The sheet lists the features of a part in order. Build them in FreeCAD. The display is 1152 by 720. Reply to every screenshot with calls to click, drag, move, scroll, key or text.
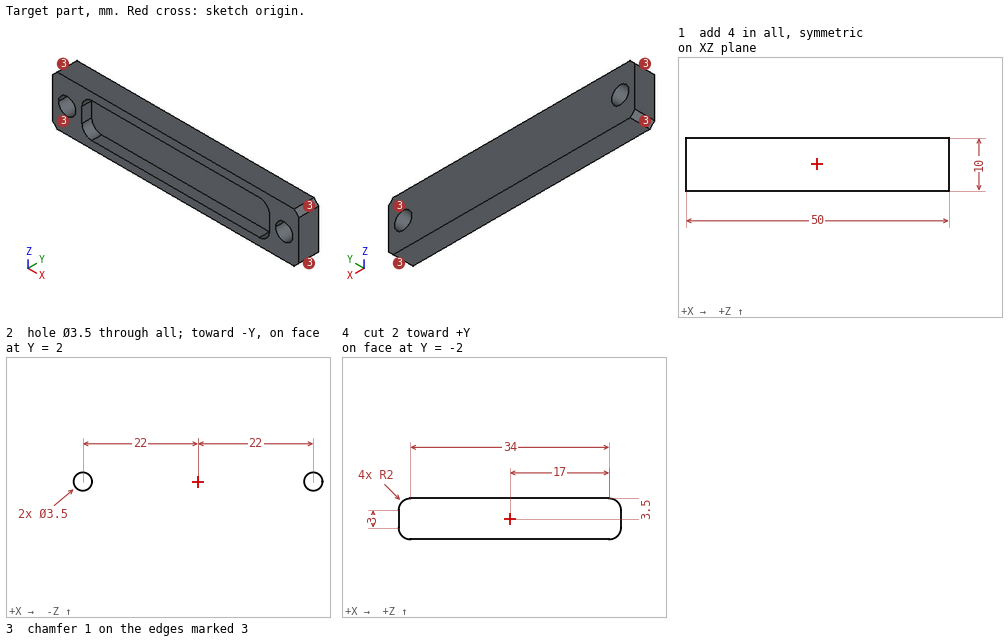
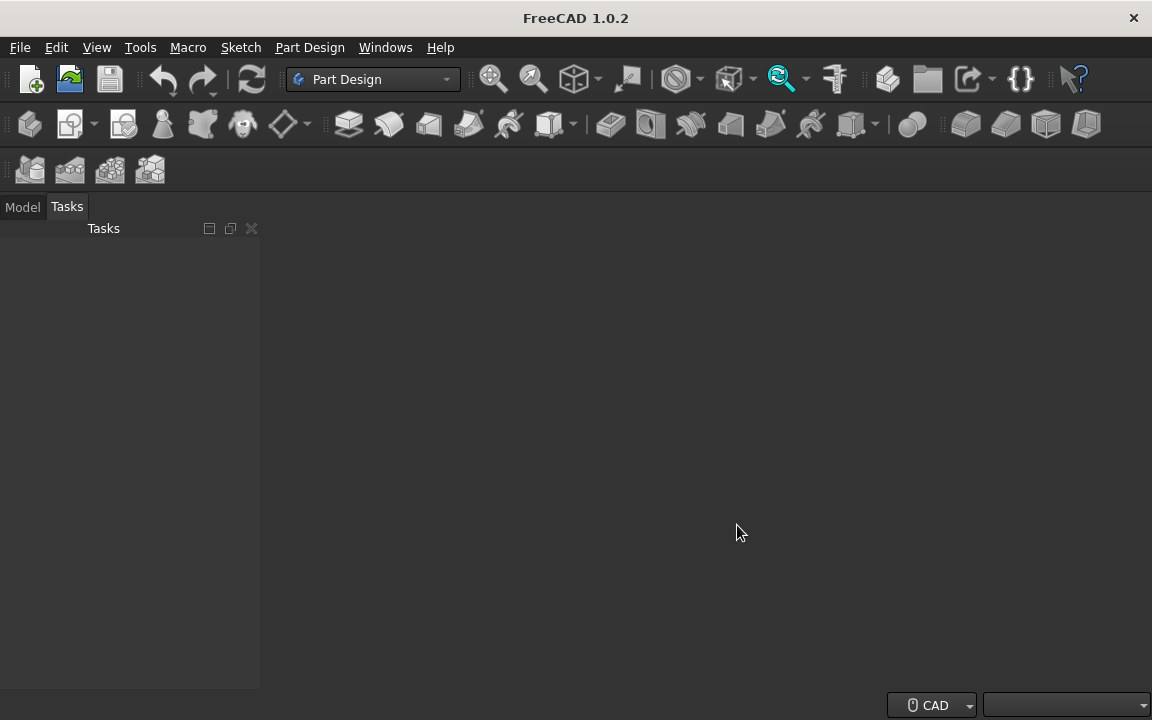
click(30, 80)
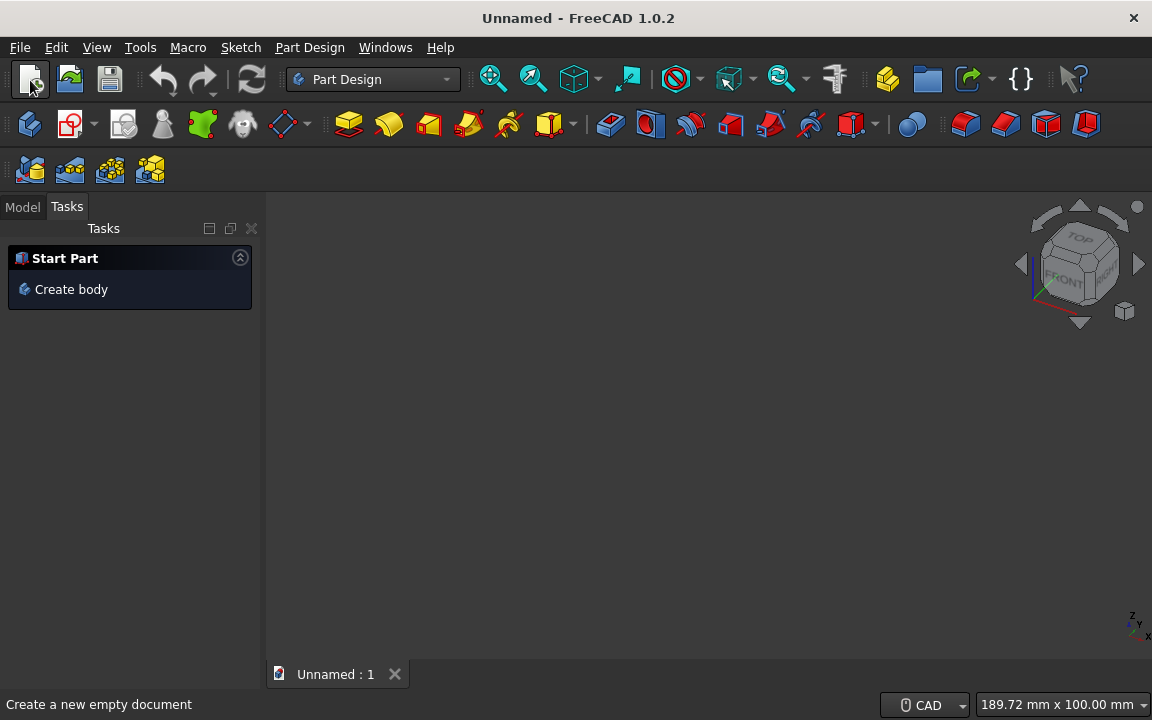
click(70, 124)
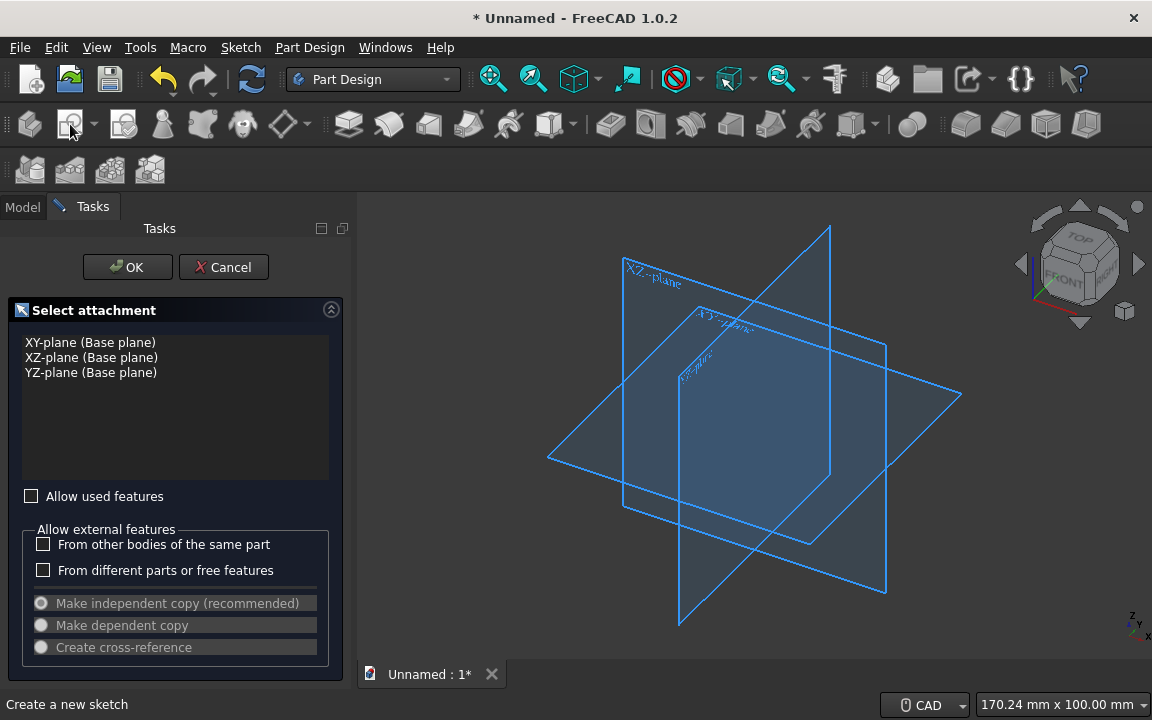
click(82, 358)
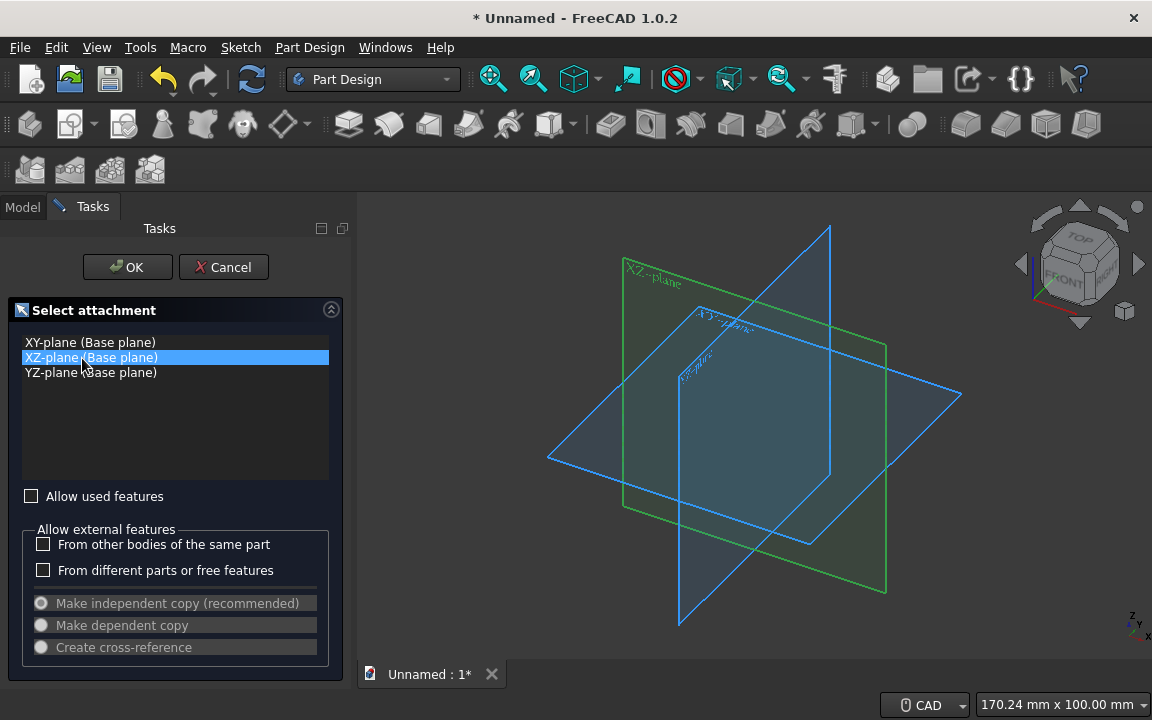
click(128, 267)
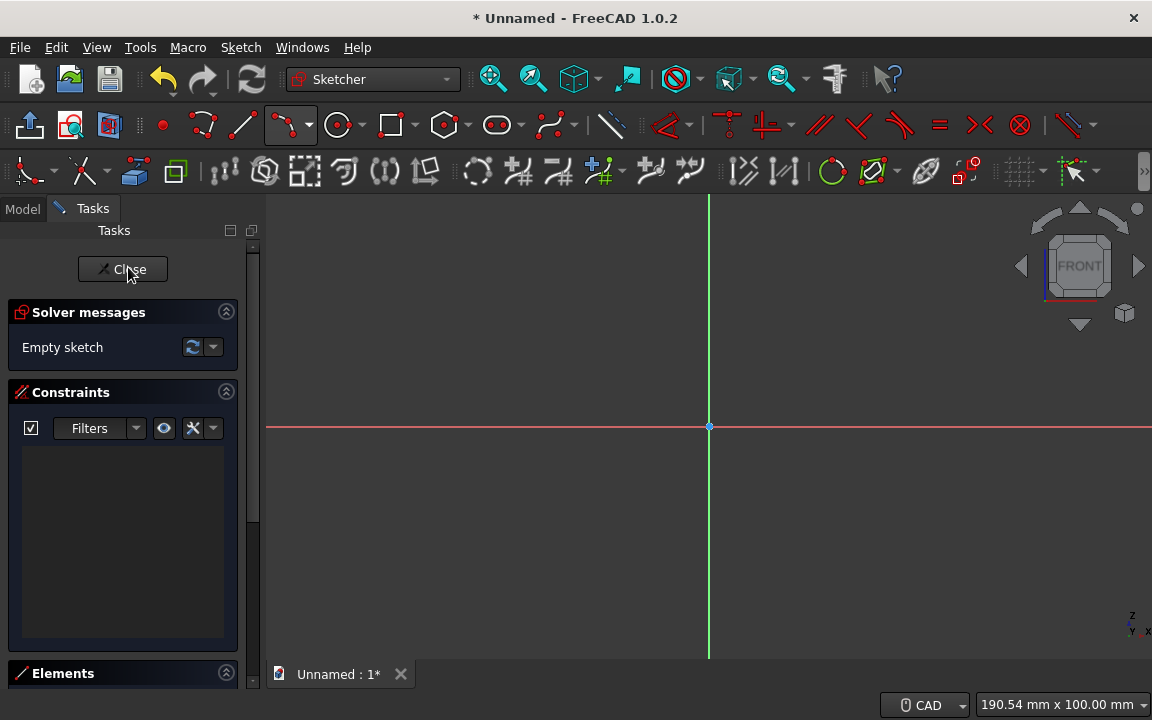
scroll(765, 426, up, 4)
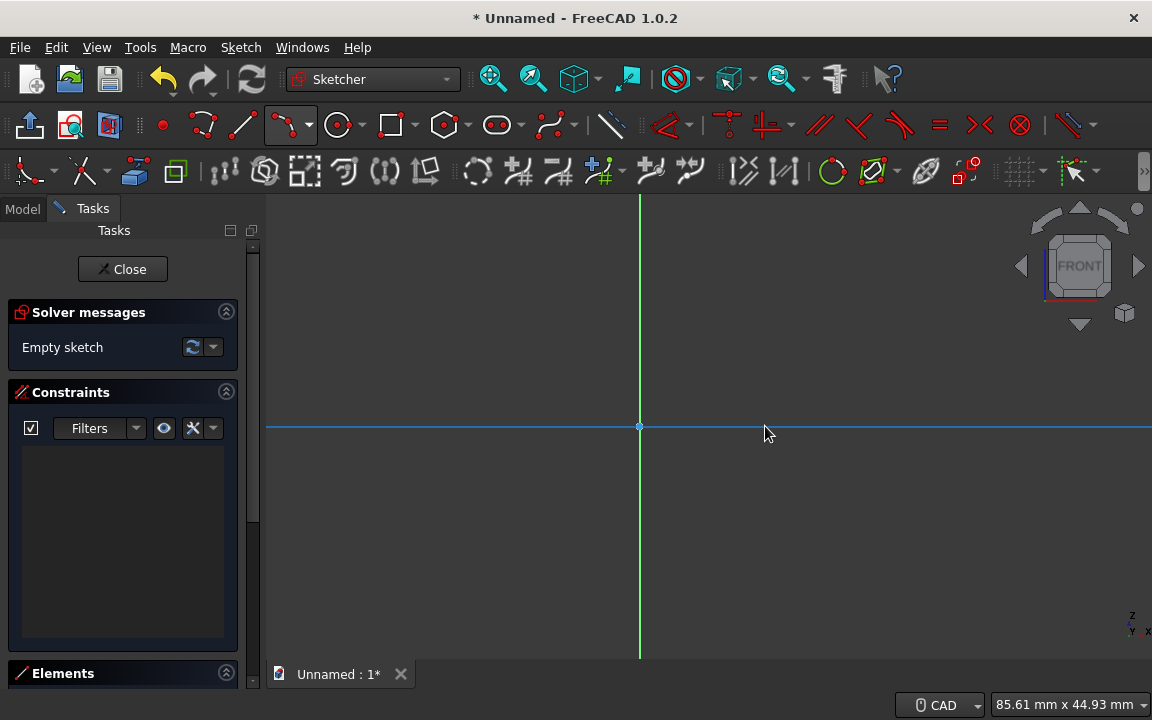
click(418, 126)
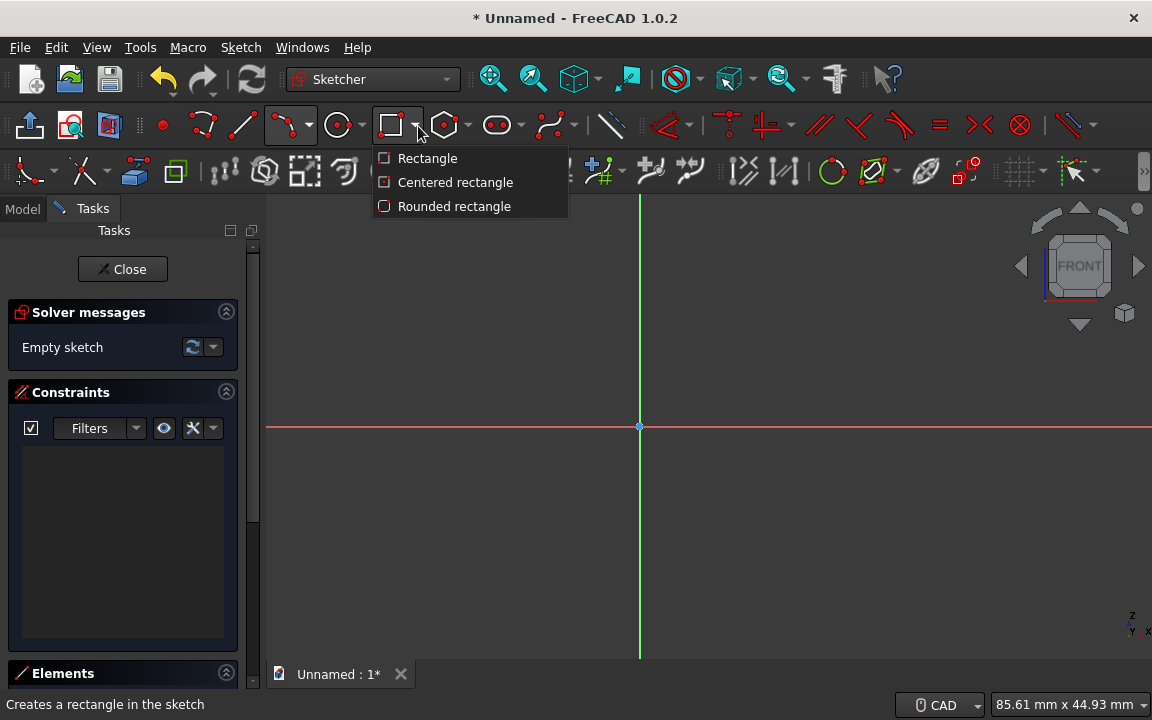
click(470, 182)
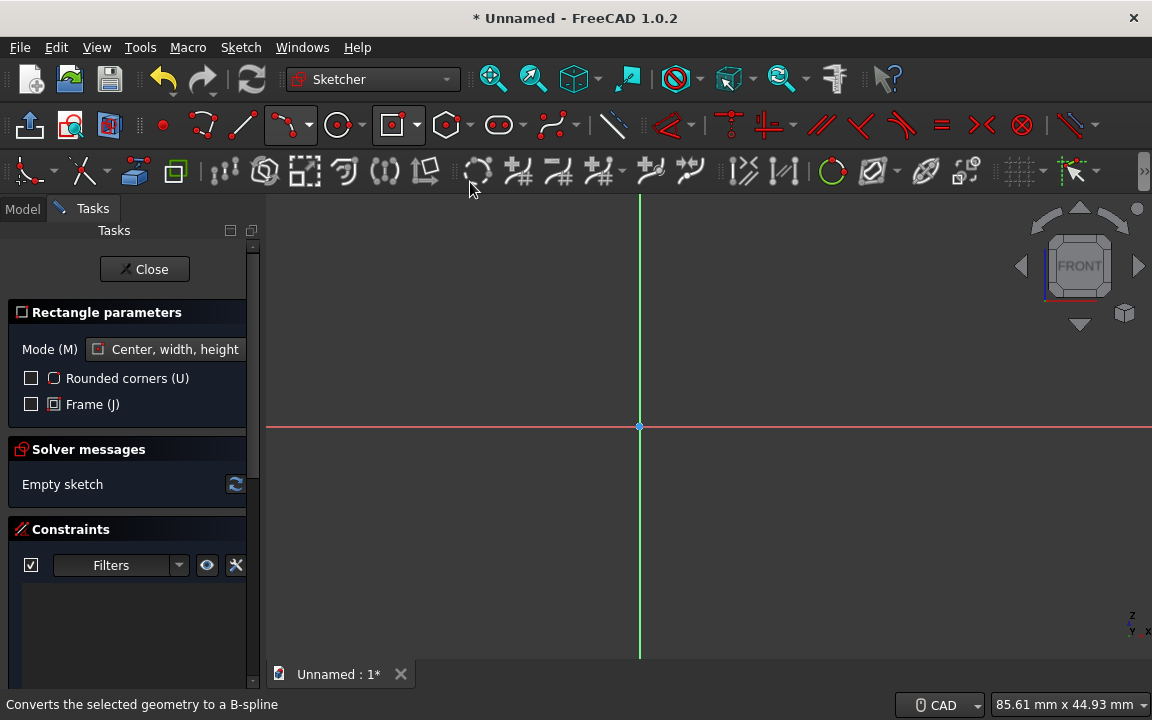
click(640, 426)
click(898, 375)
key(Escape)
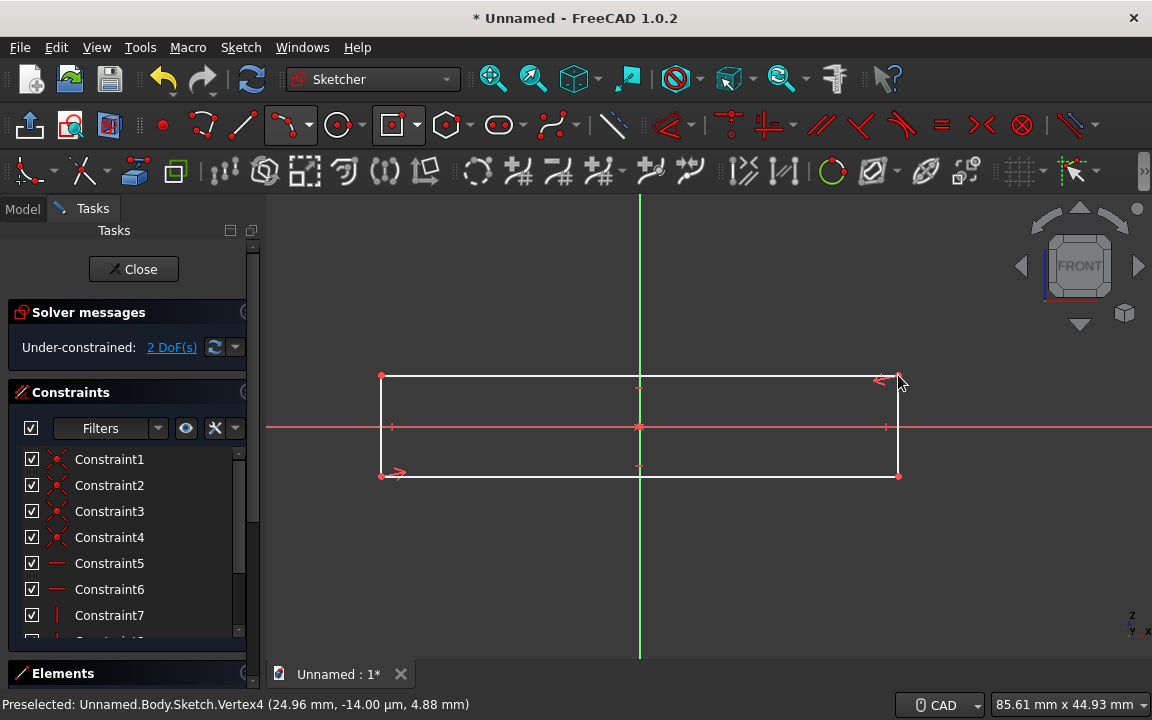
click(536, 477)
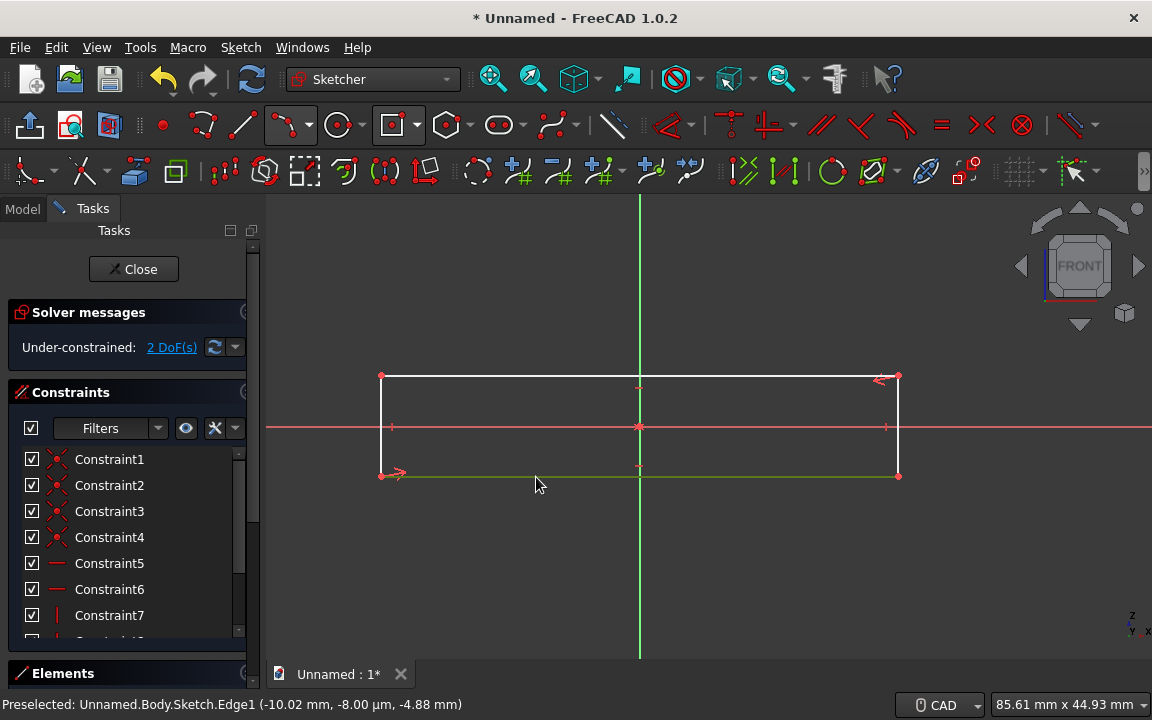
key(l)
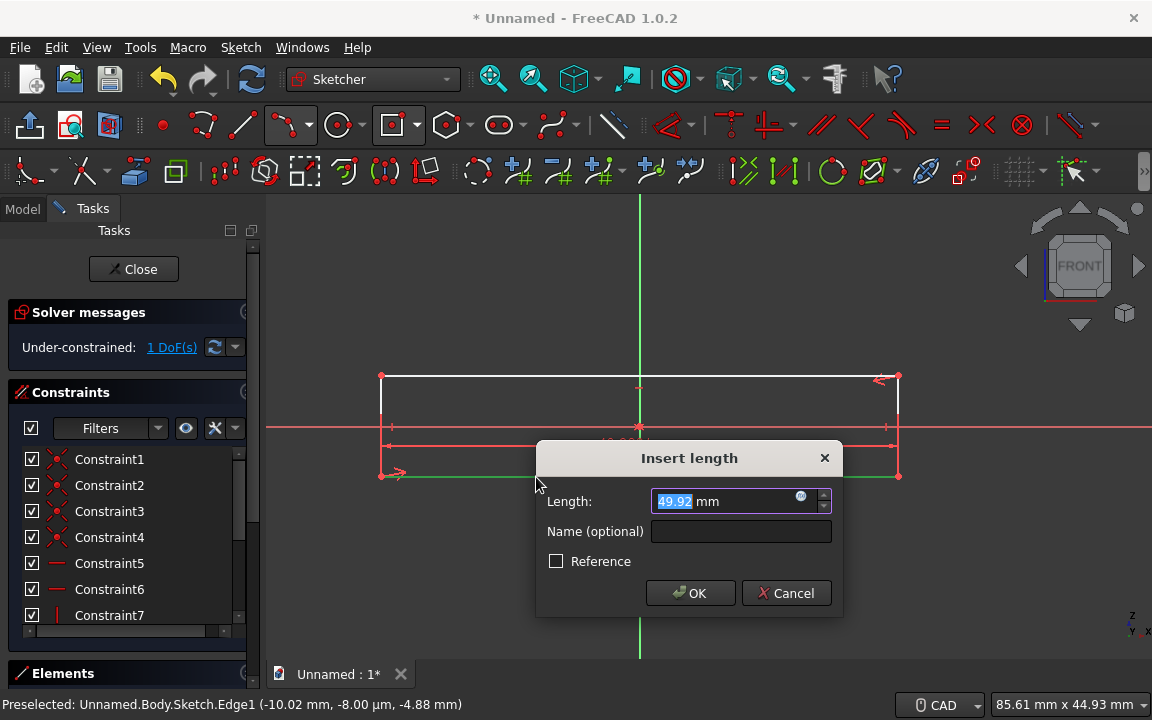
text(50)
key(Return)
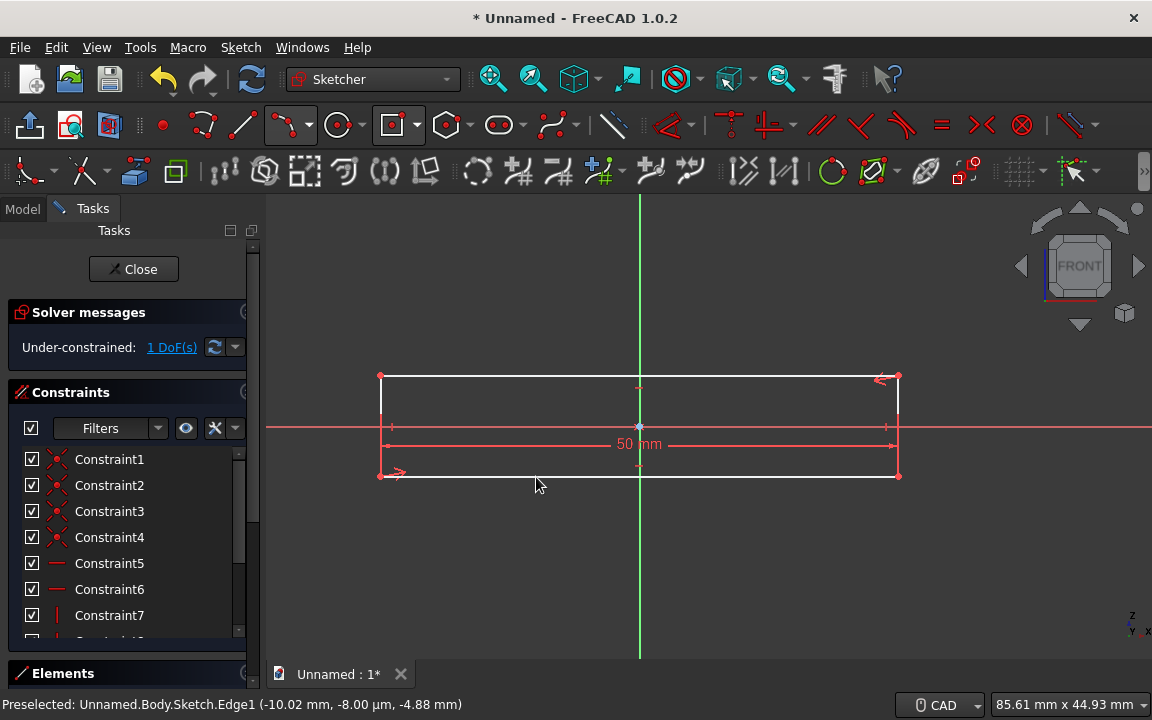
click(898, 447)